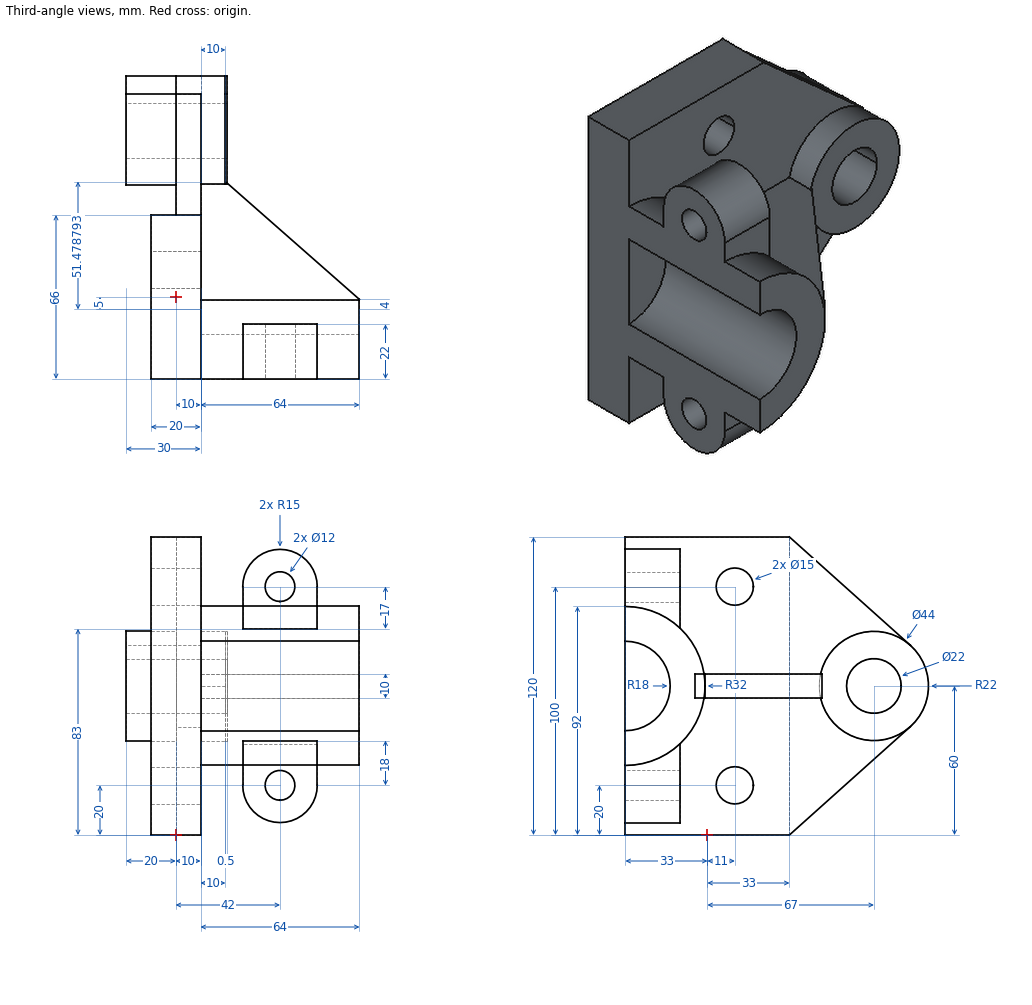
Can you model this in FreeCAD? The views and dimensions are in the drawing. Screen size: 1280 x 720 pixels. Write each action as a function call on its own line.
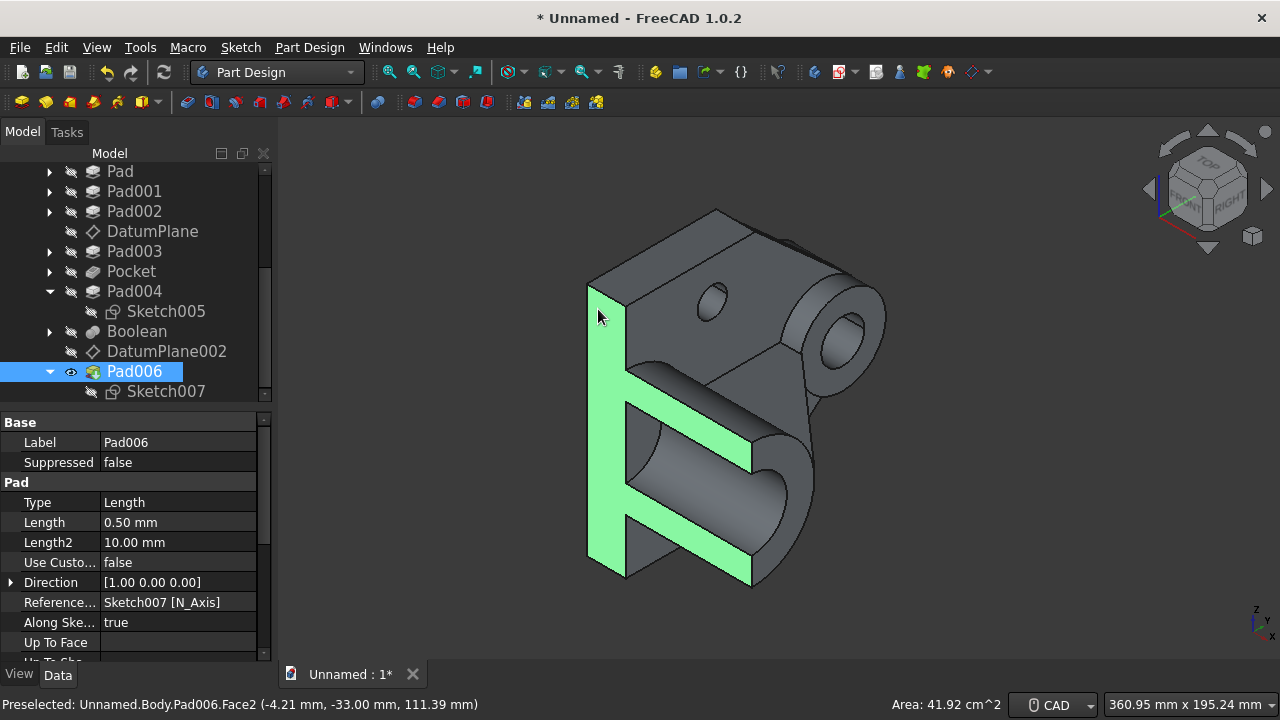
click(840, 72)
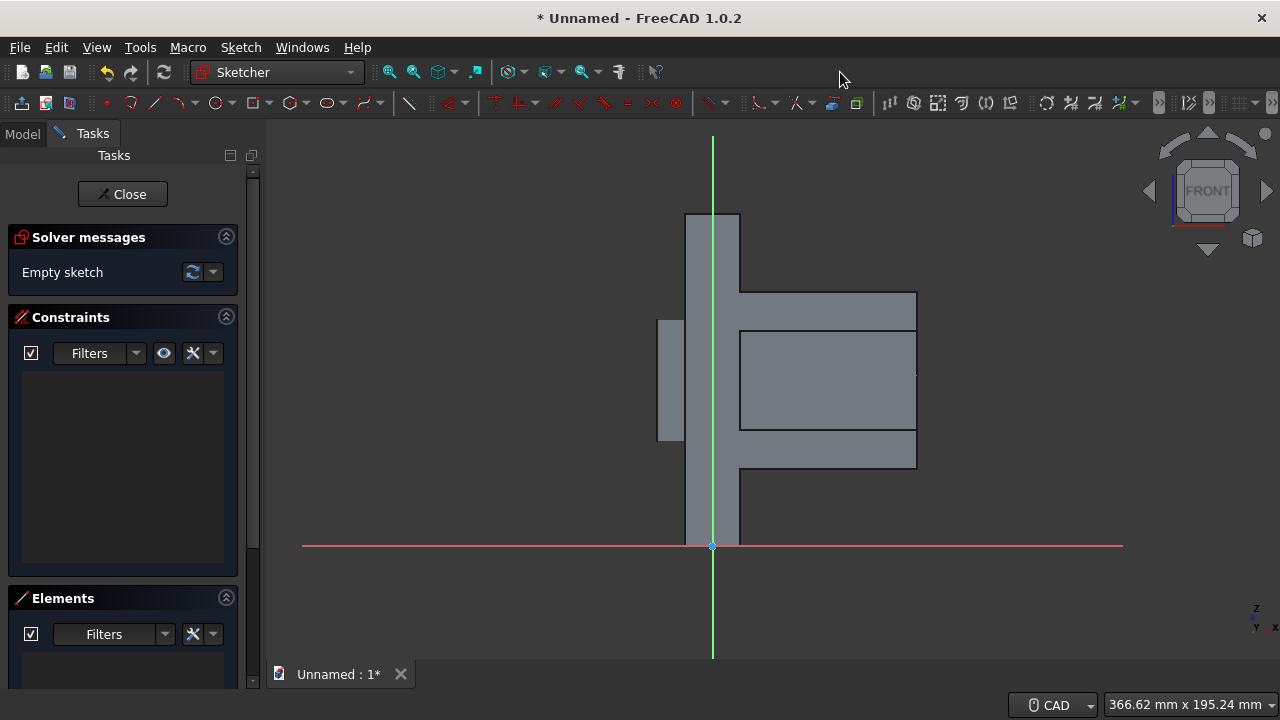
click(132, 104)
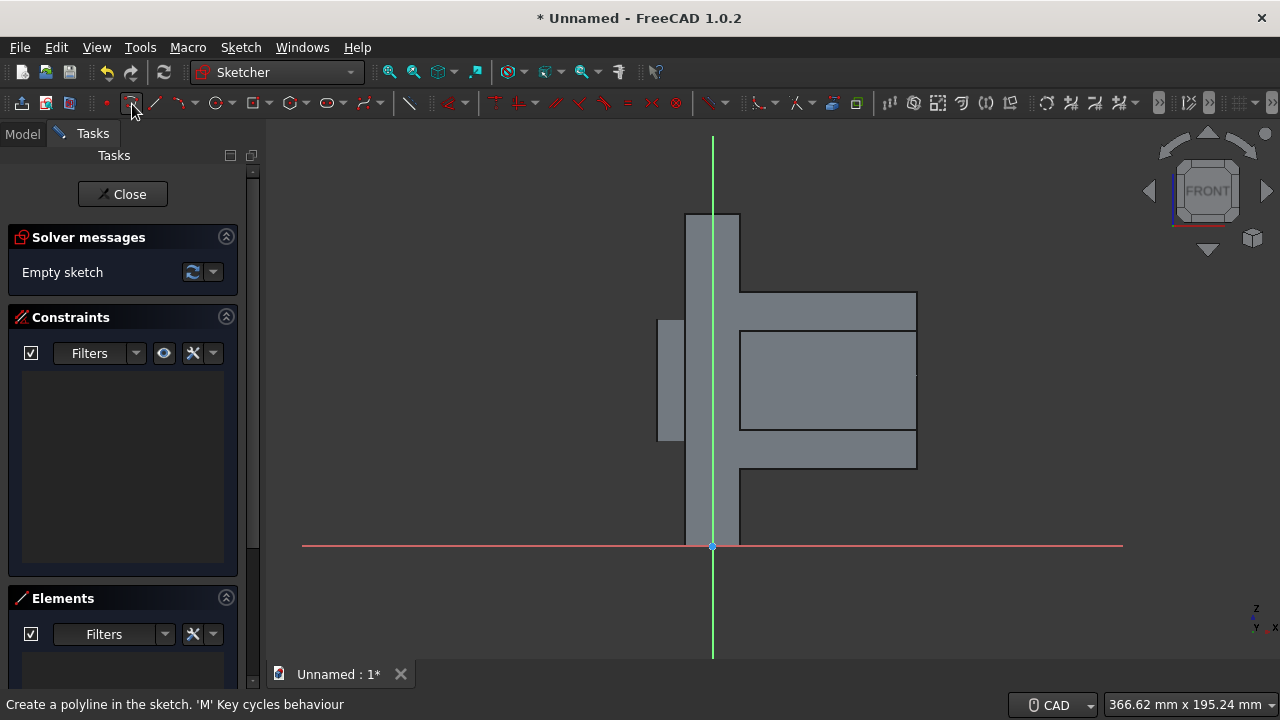
click(787, 270)
click(787, 317)
click(870, 317)
click(870, 270)
right_click(870, 270)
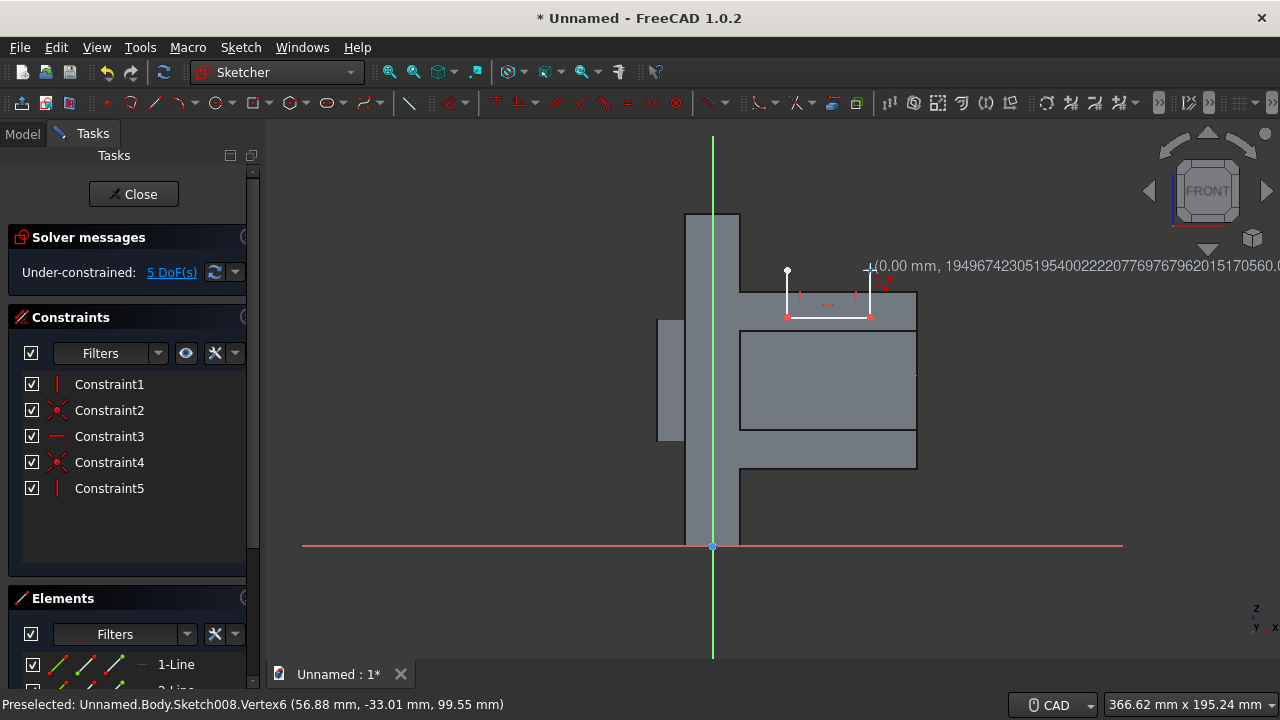
click(180, 104)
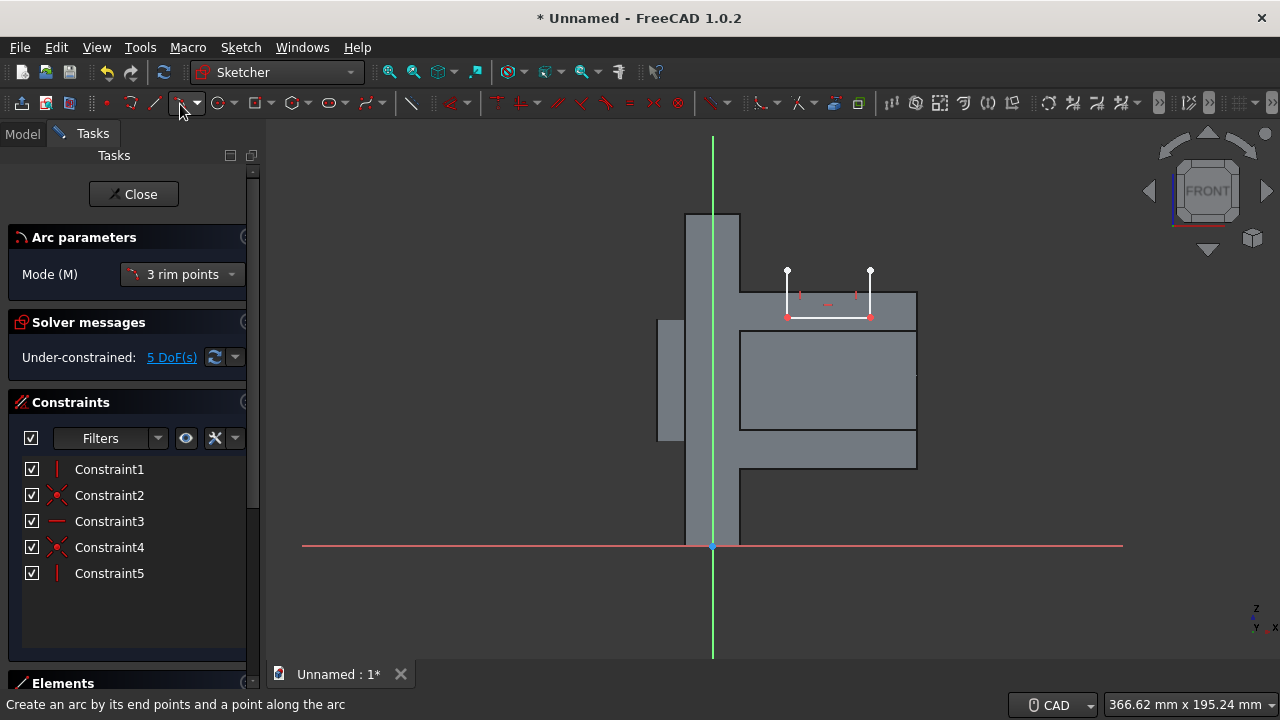
click(870, 271)
click(787, 271)
click(829, 228)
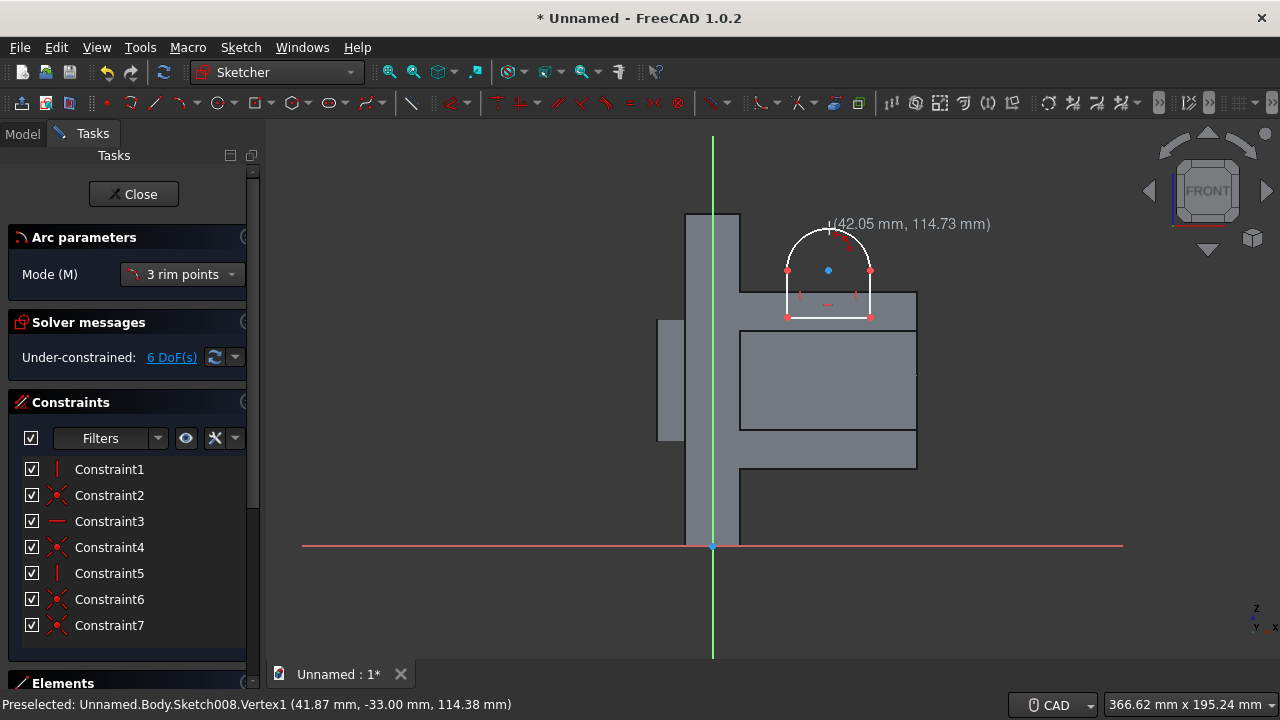
click(132, 104)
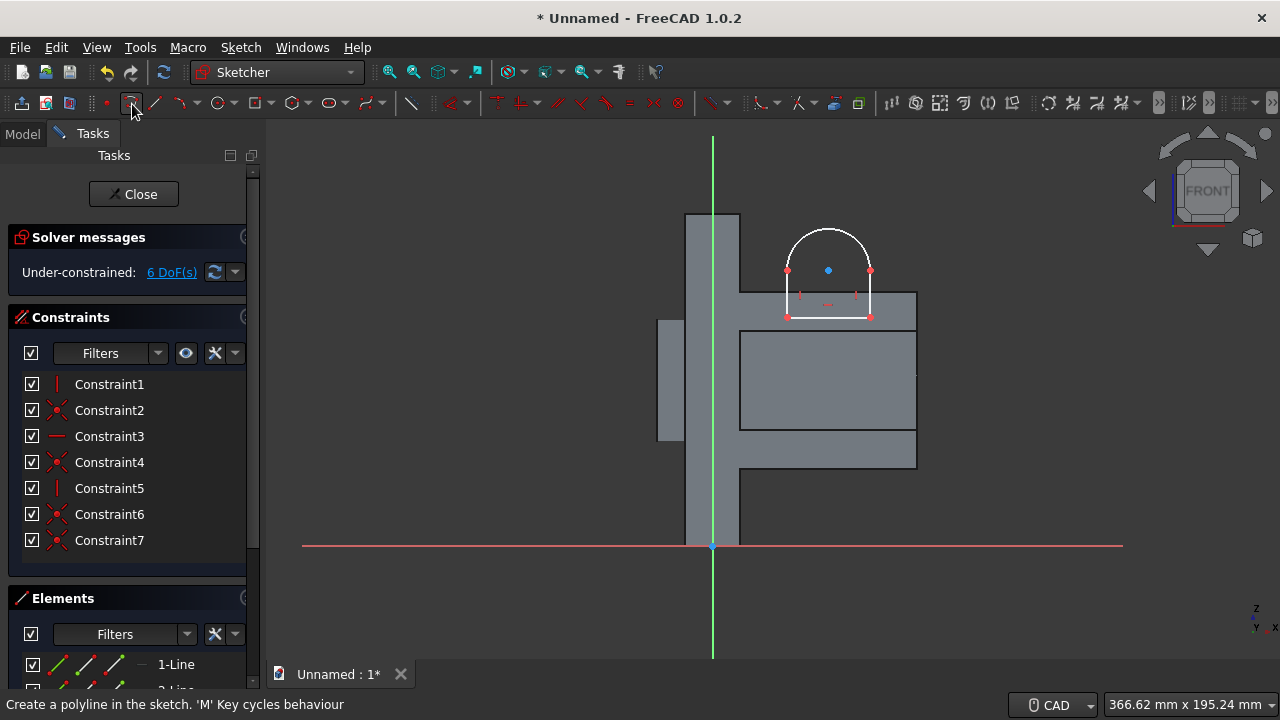
click(870, 491)
click(870, 441)
click(787, 441)
click(787, 491)
right_click(787, 491)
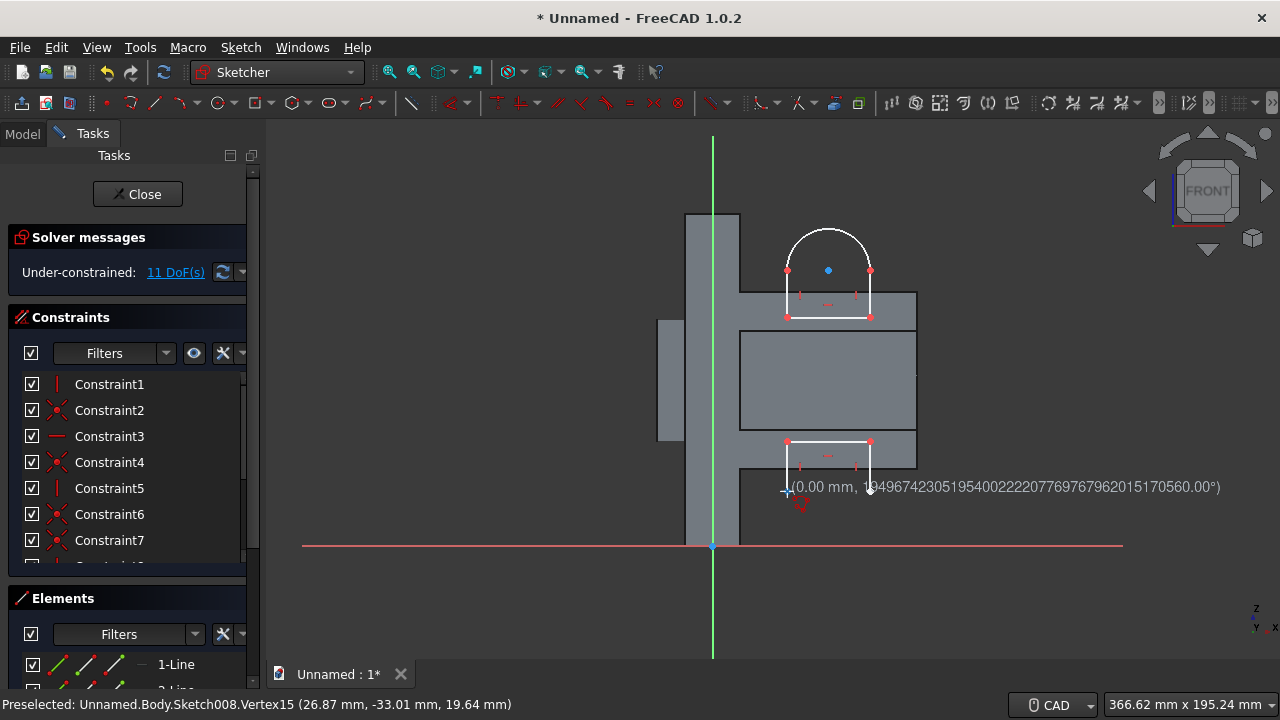
click(180, 104)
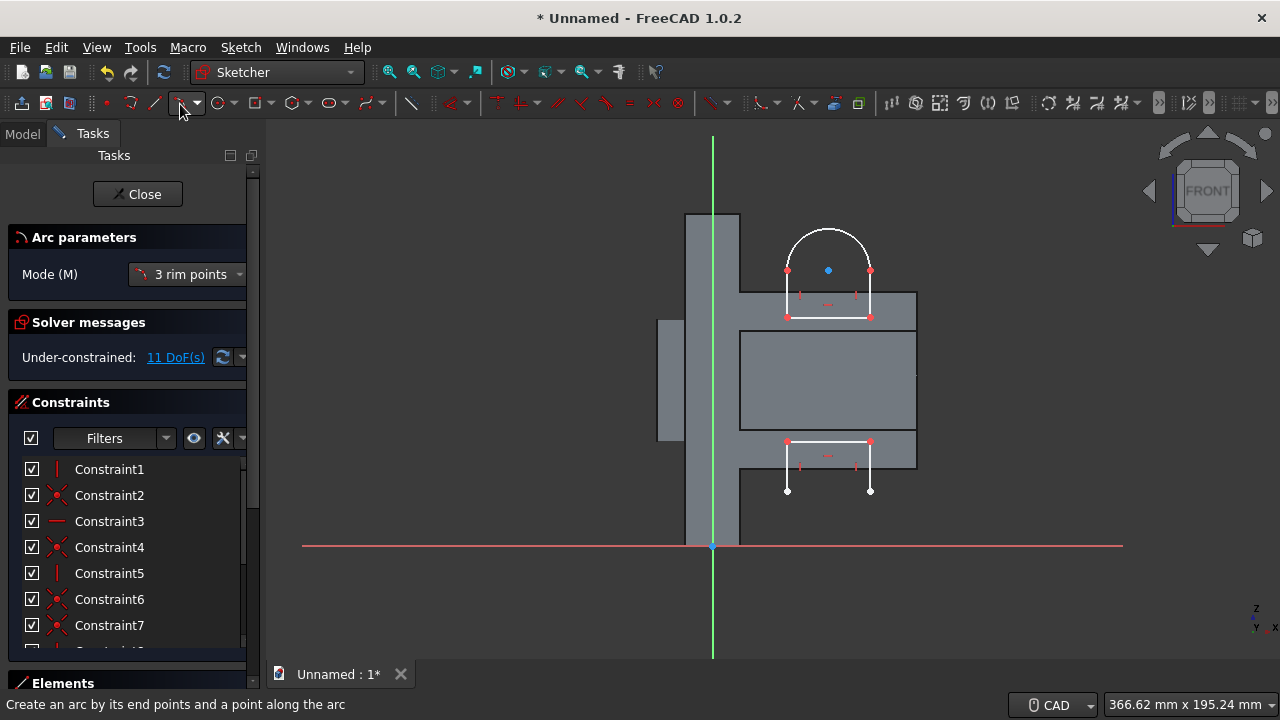
click(787, 492)
click(870, 492)
click(816, 530)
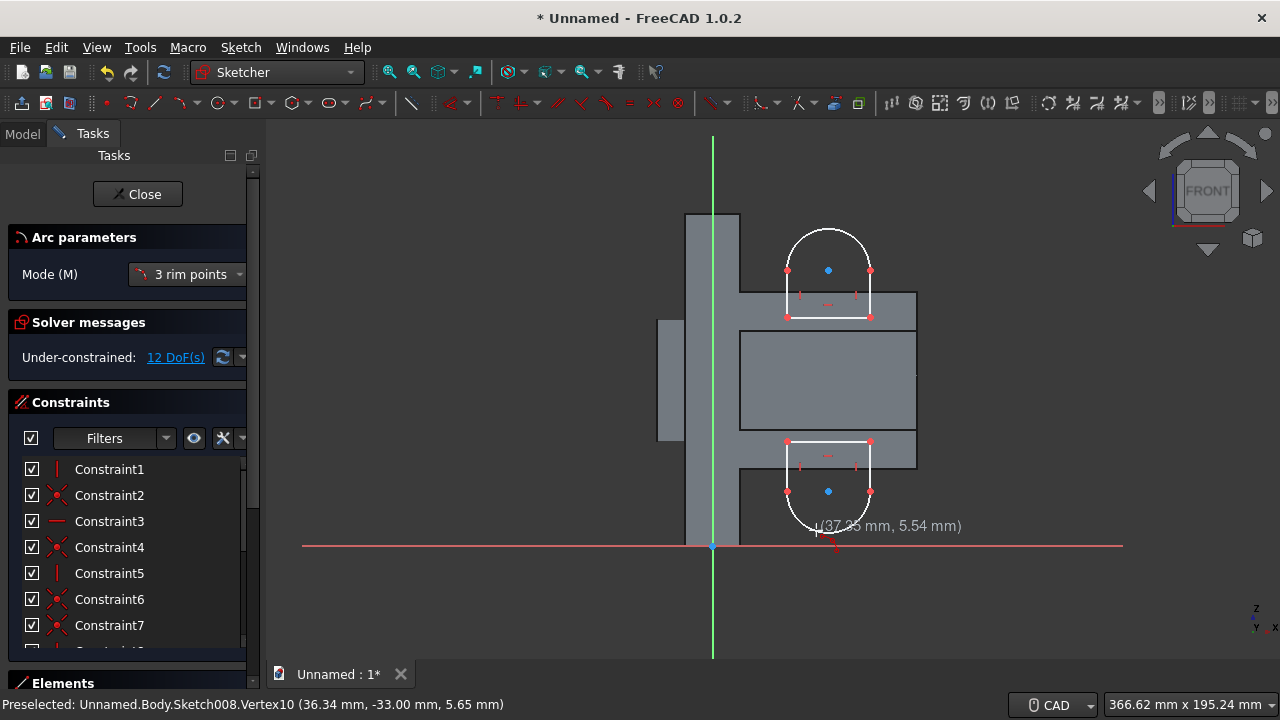
click(218, 104)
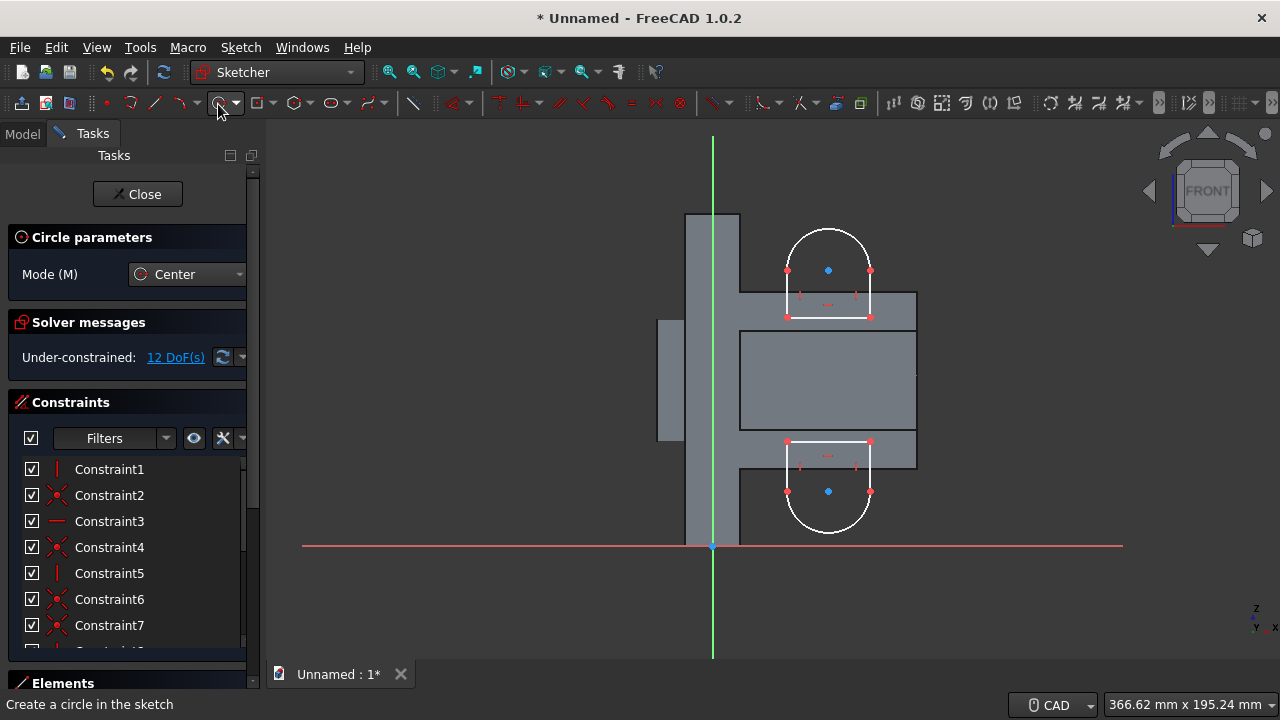
scroll(829, 270, up, 2)